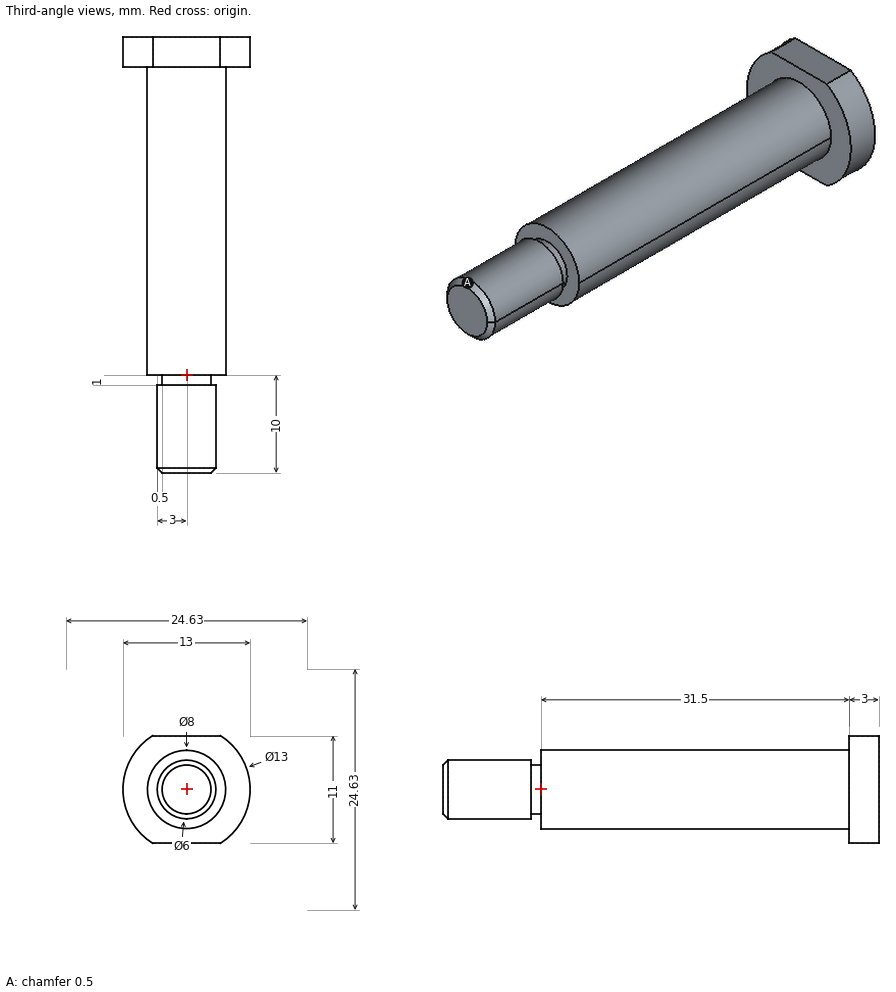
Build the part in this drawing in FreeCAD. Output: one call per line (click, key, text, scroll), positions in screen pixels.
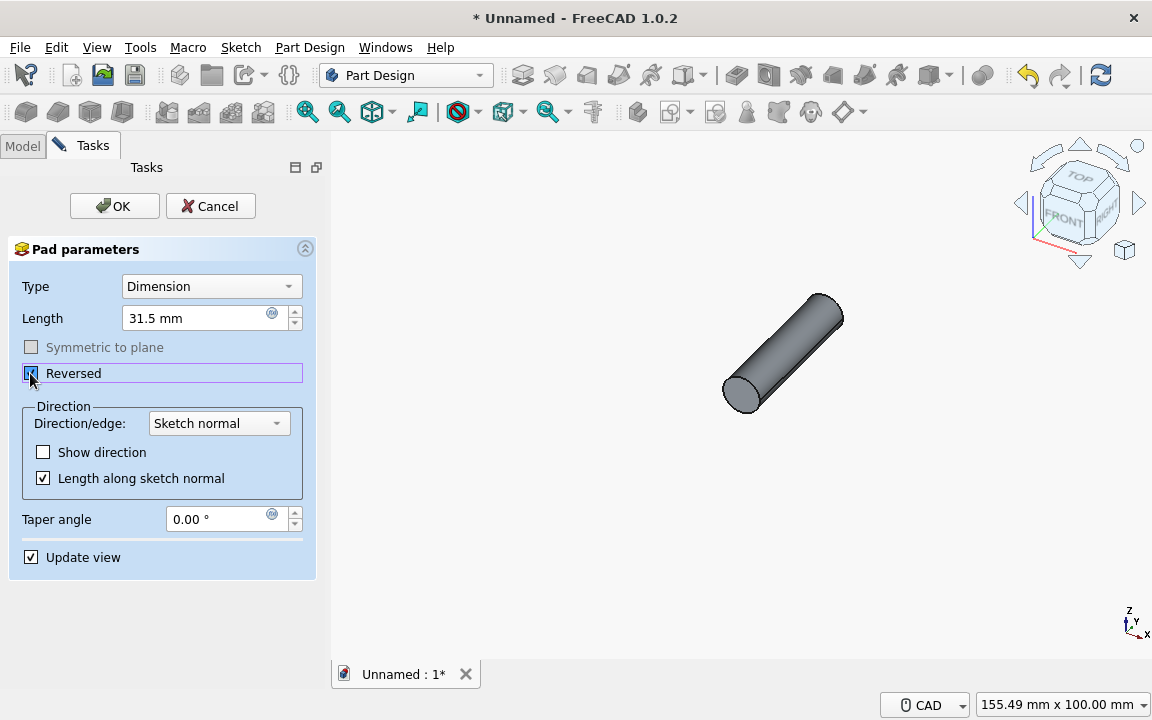
click(115, 206)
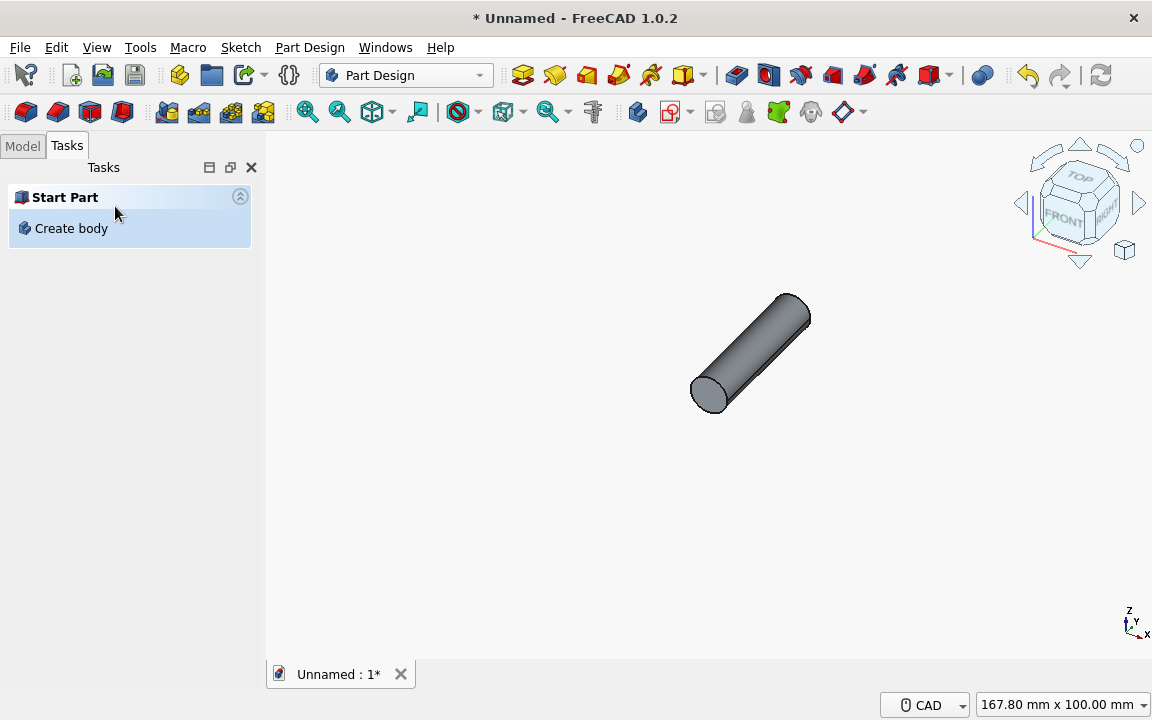
key(v)
key(f)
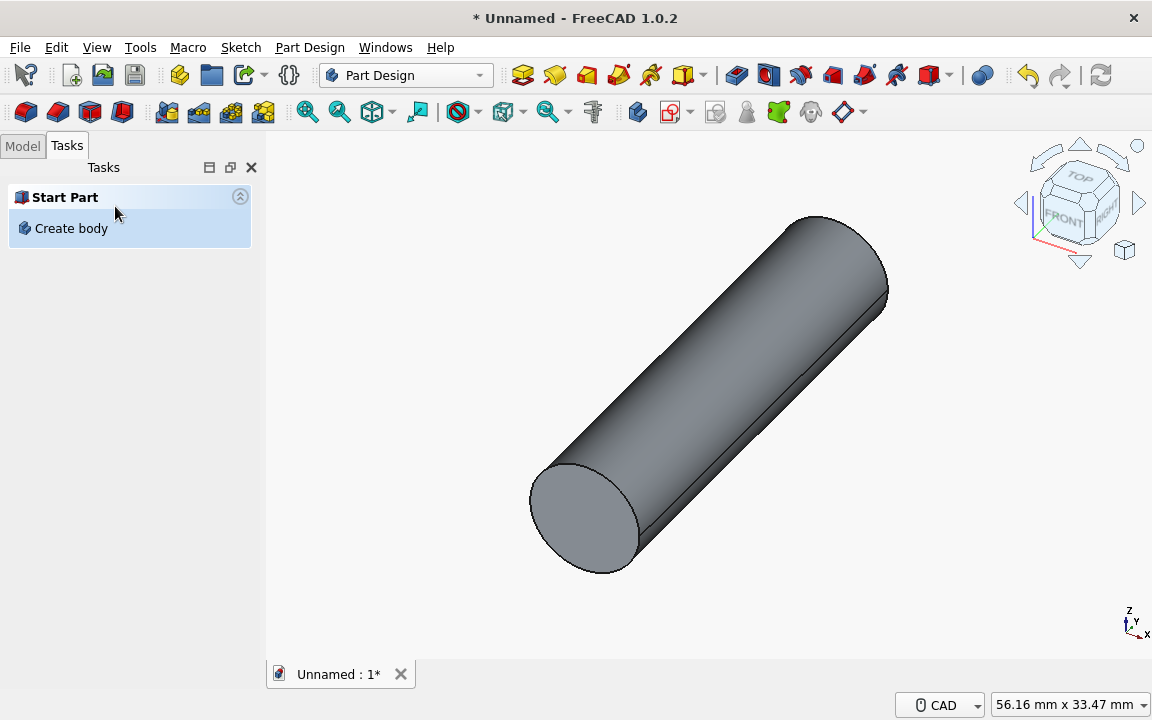
click(585, 517)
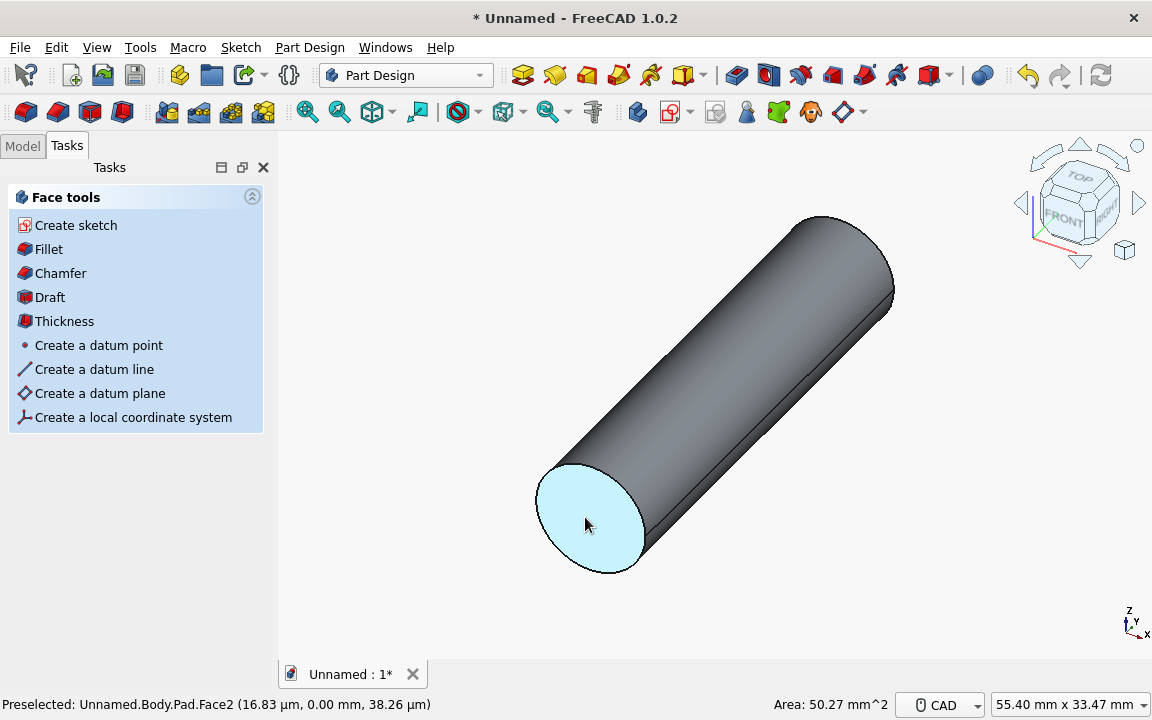
click(670, 112)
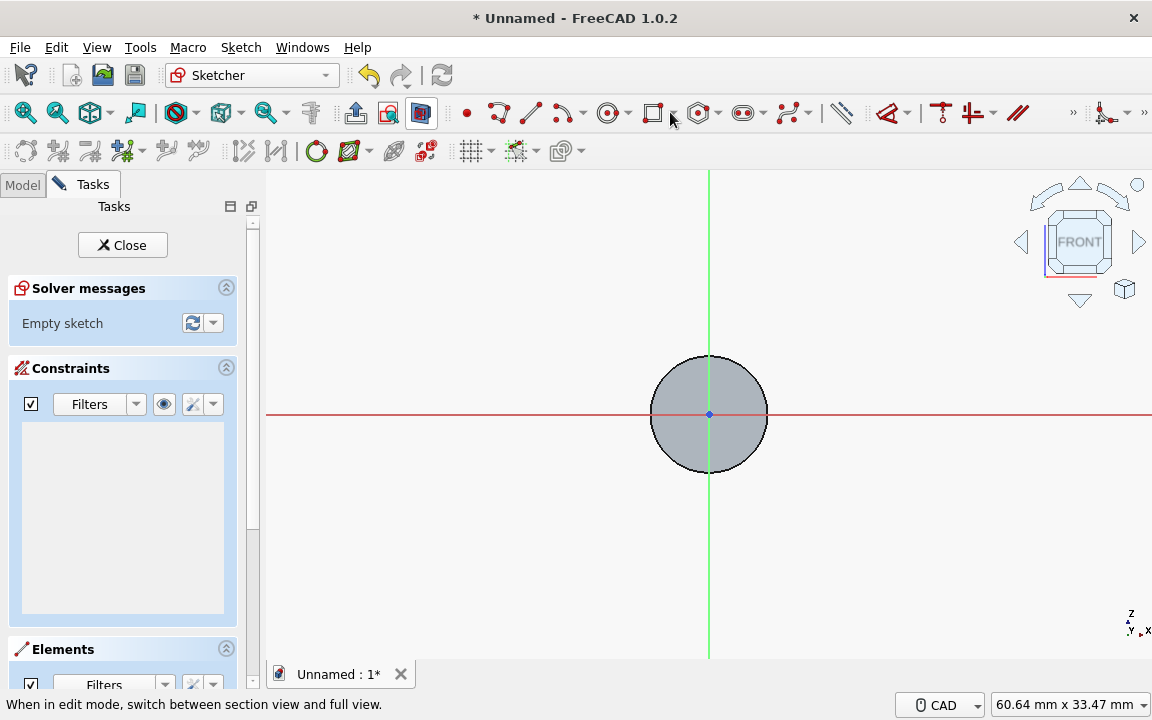
scroll(739, 415, up, 6)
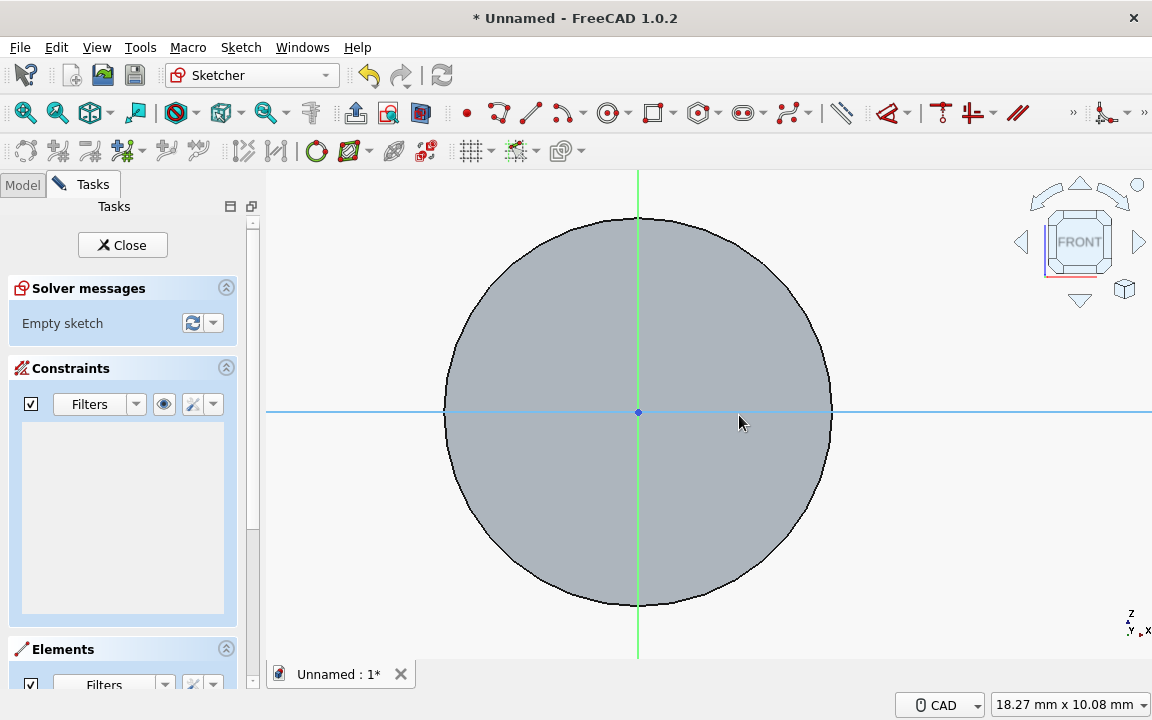
click(608, 114)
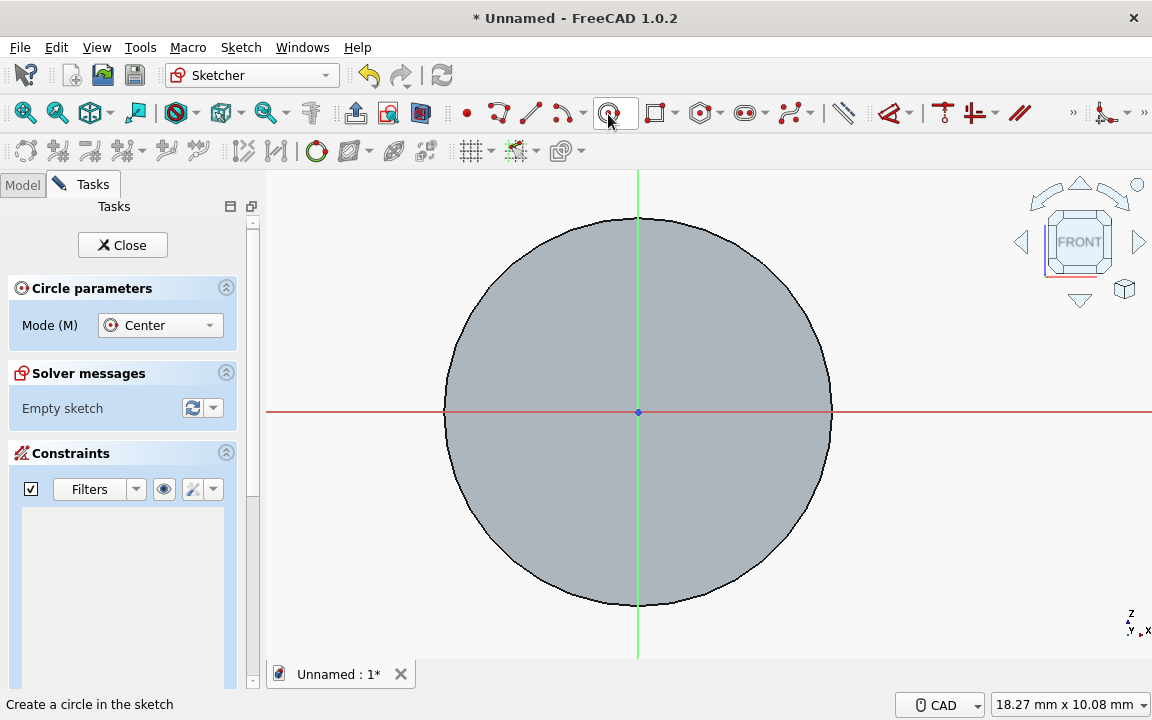
click(638, 412)
move(741, 309)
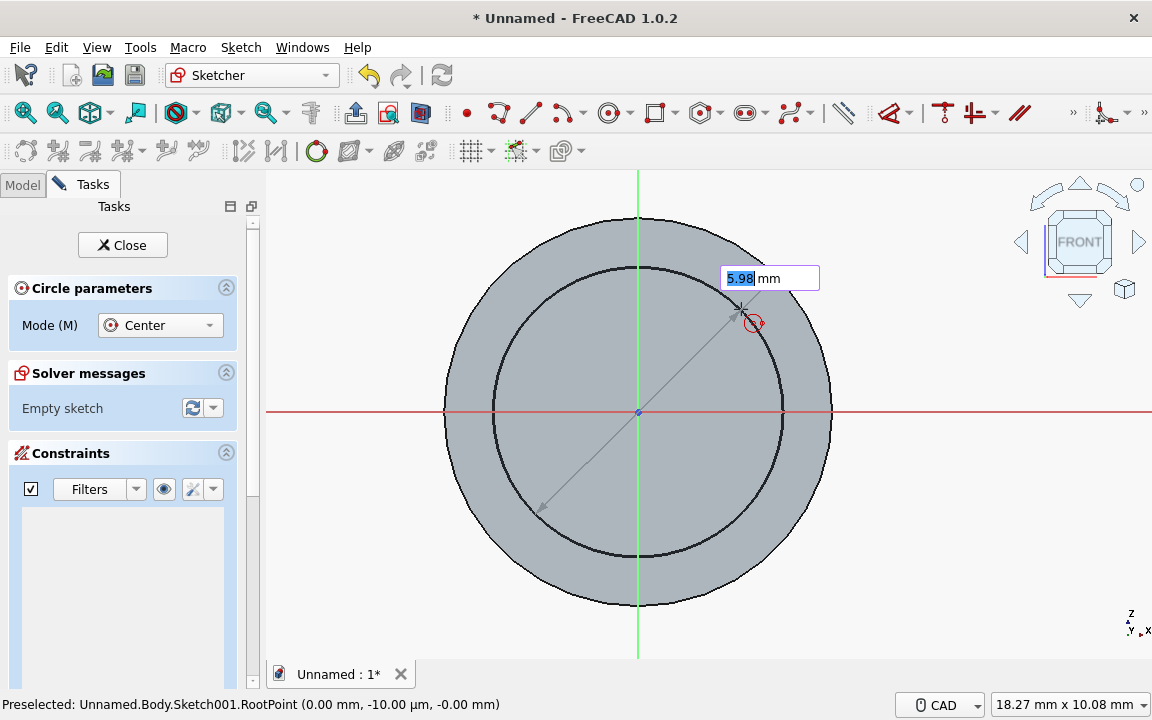
text(6)
key(Return)
key(Escape)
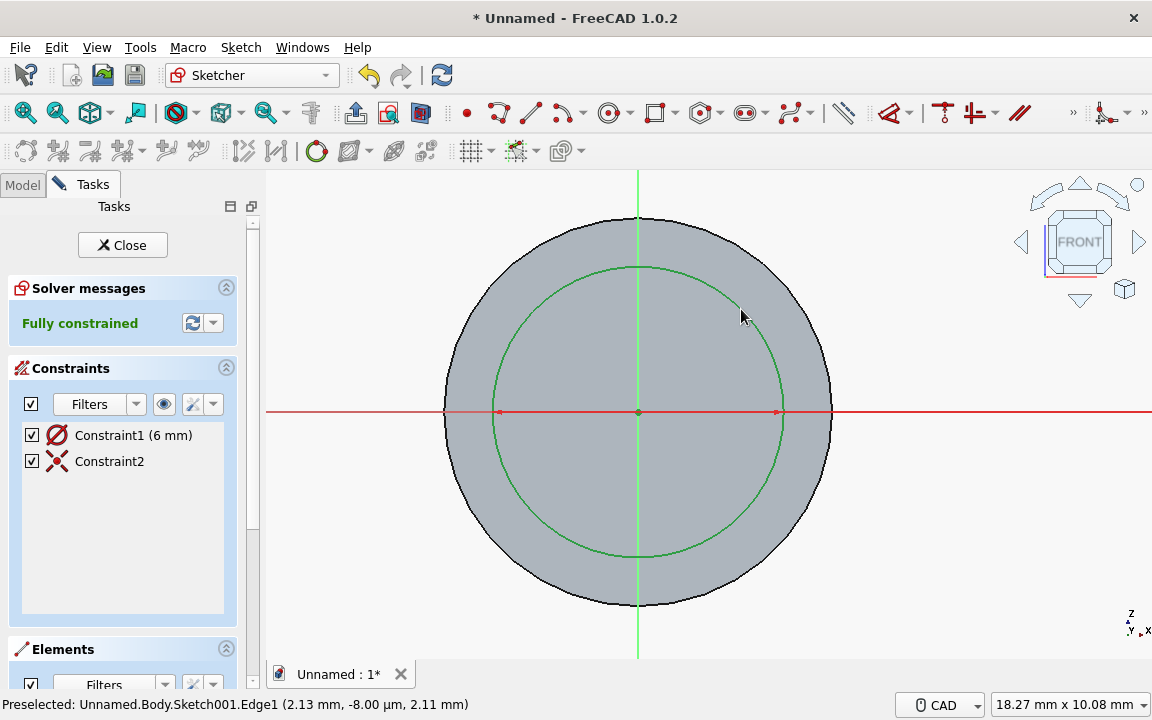
click(123, 245)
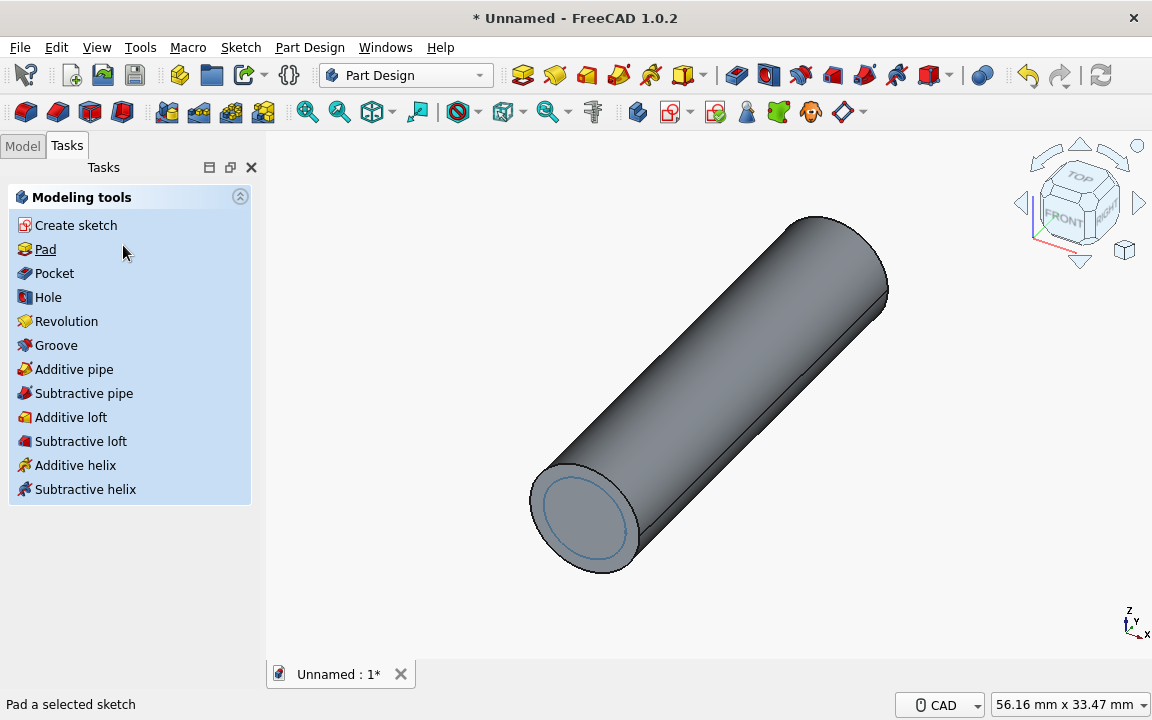
click(524, 76)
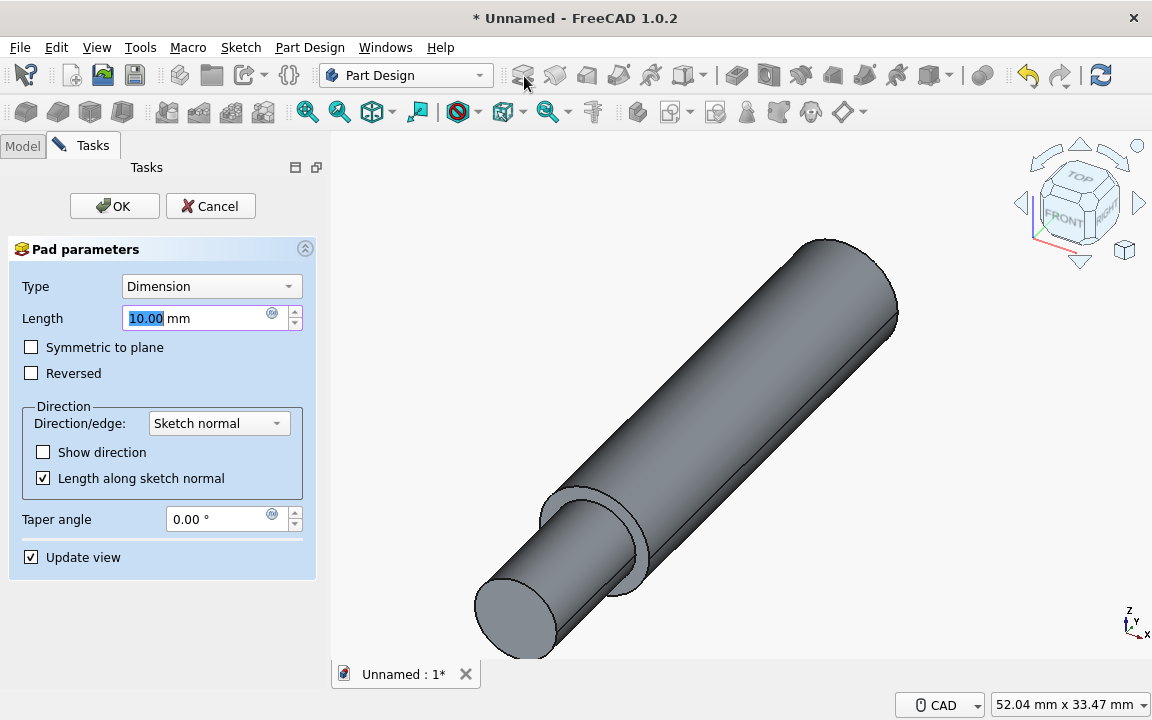
text(10)
key(Tab)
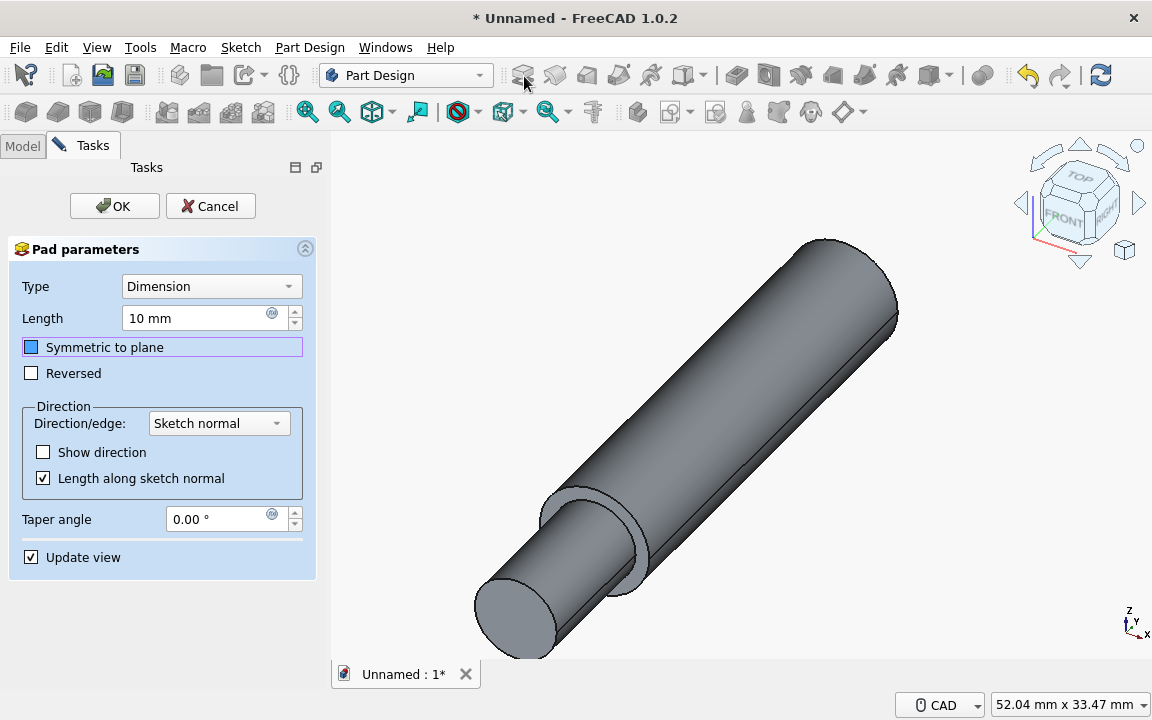
click(115, 206)